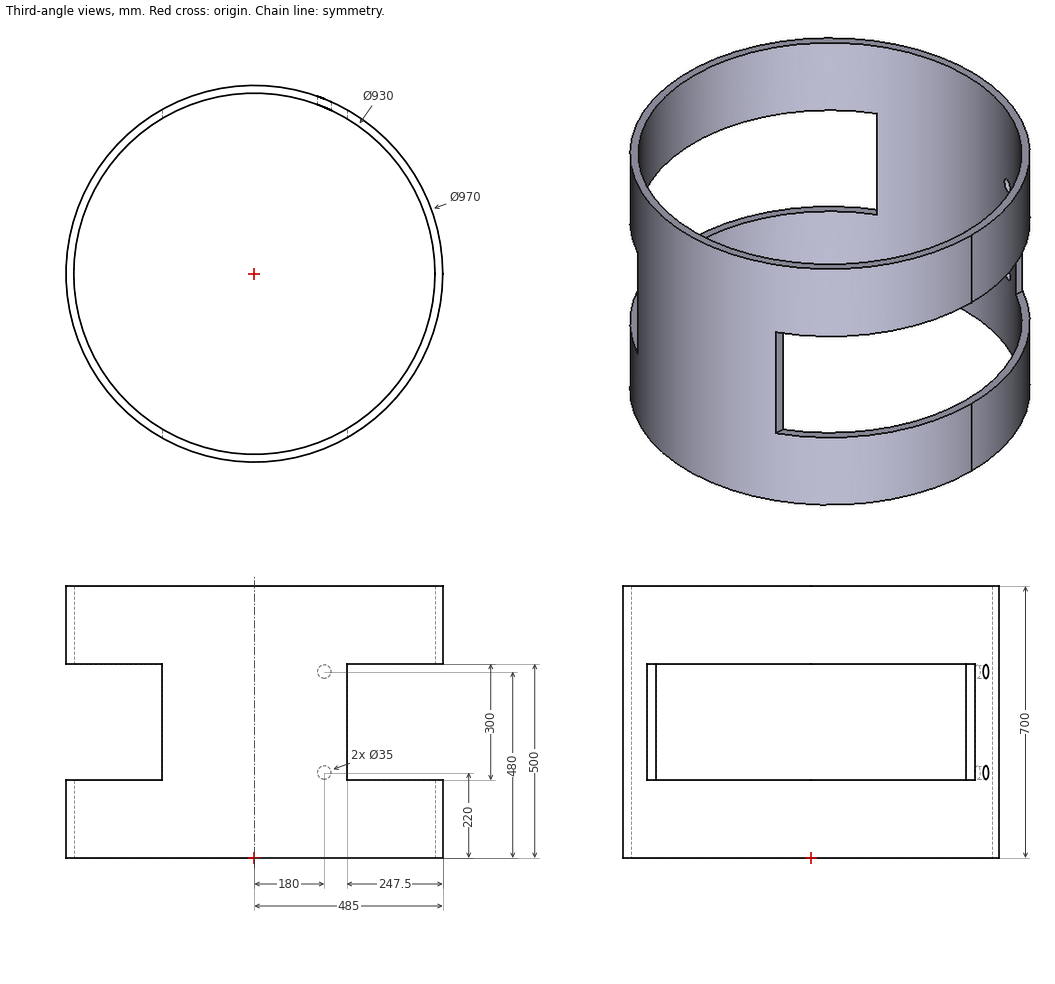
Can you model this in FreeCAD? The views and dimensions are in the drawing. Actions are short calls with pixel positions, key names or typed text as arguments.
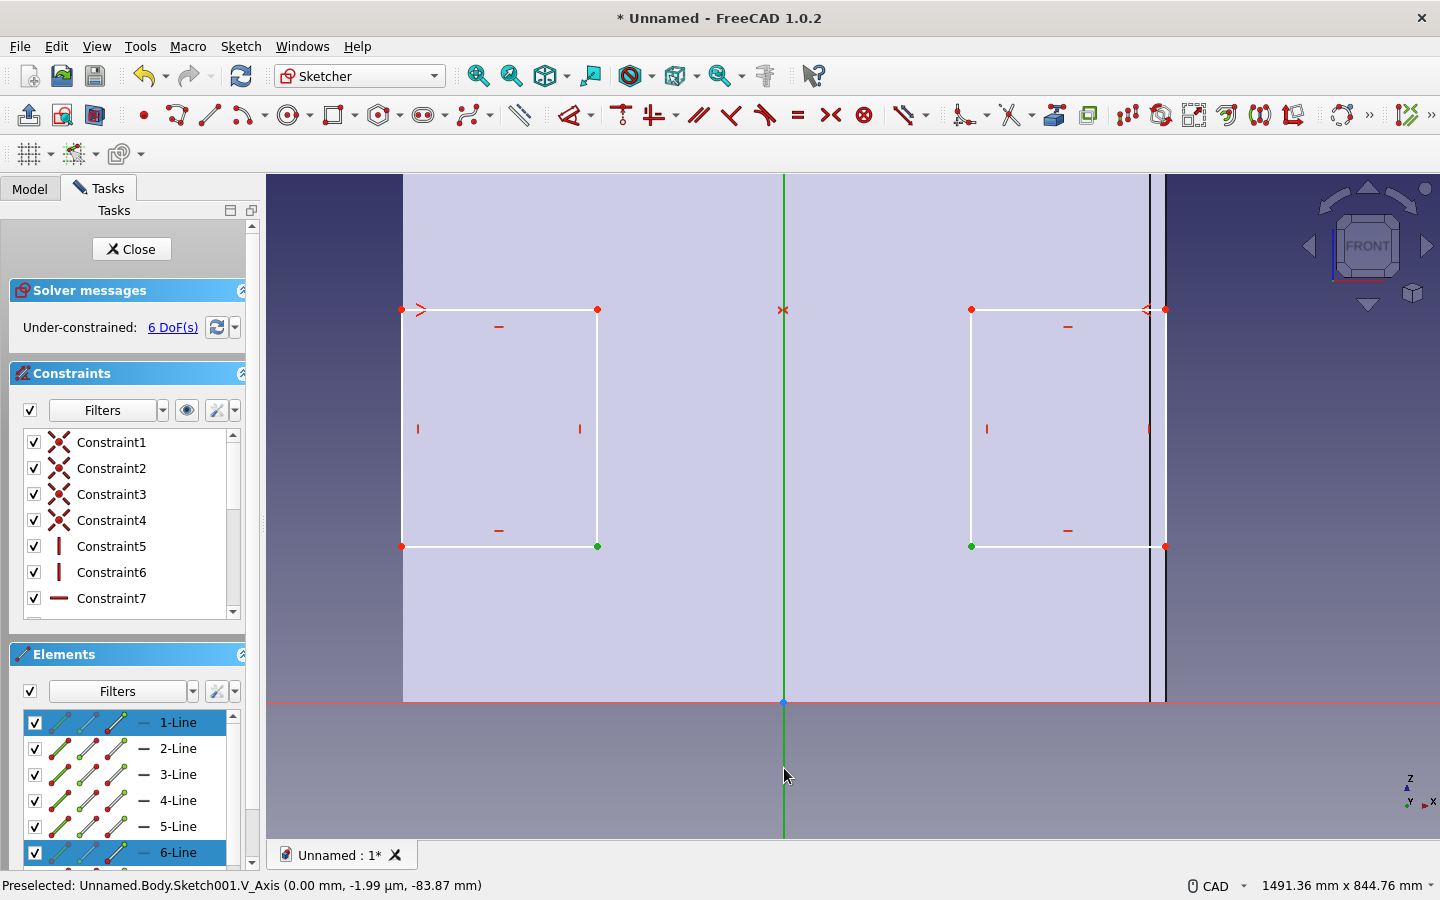
key(s)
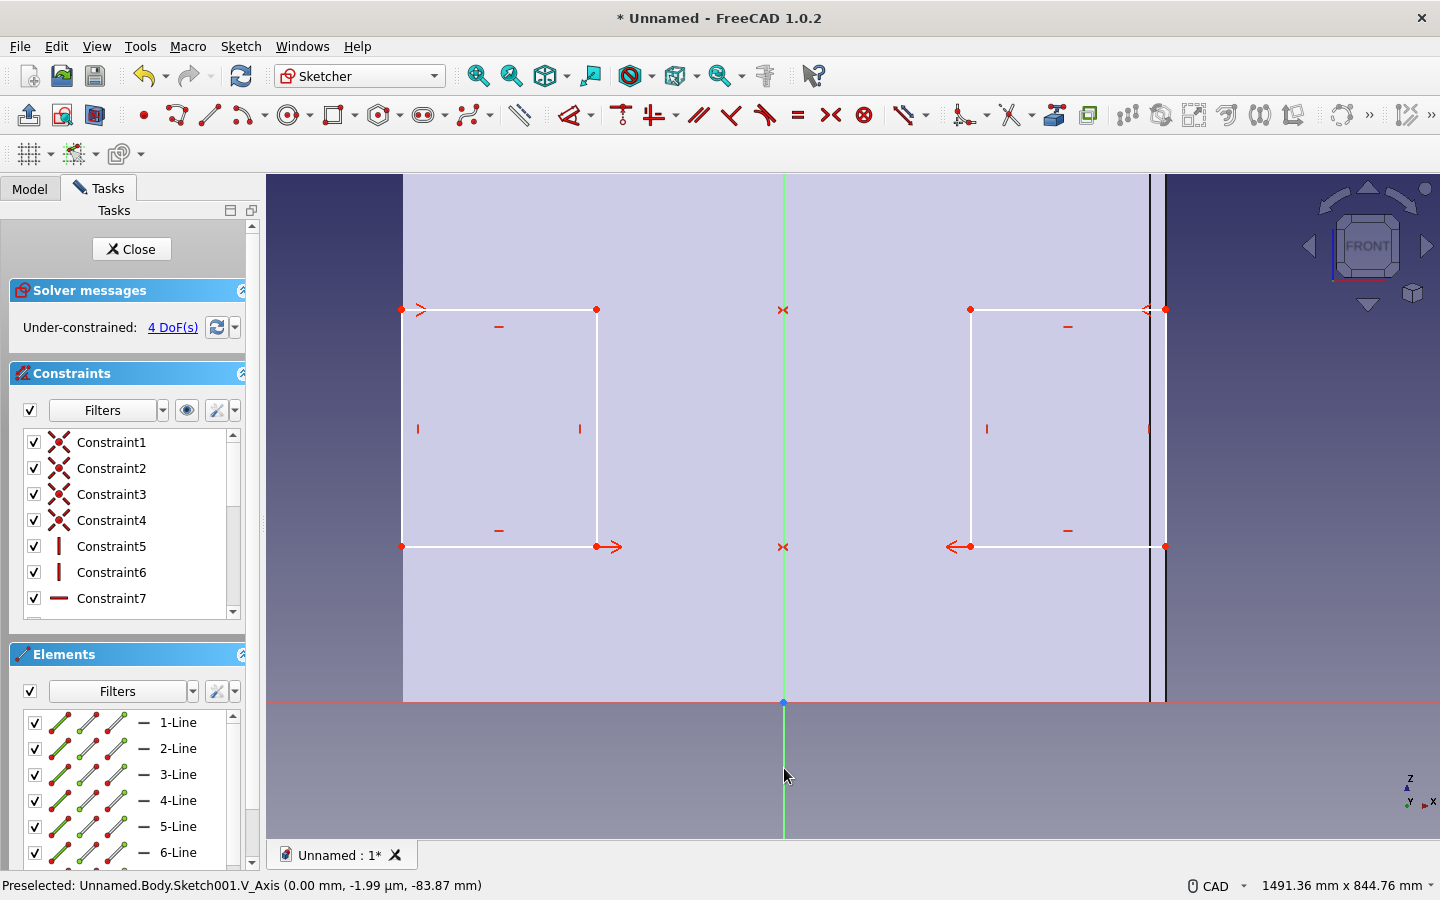
key(d)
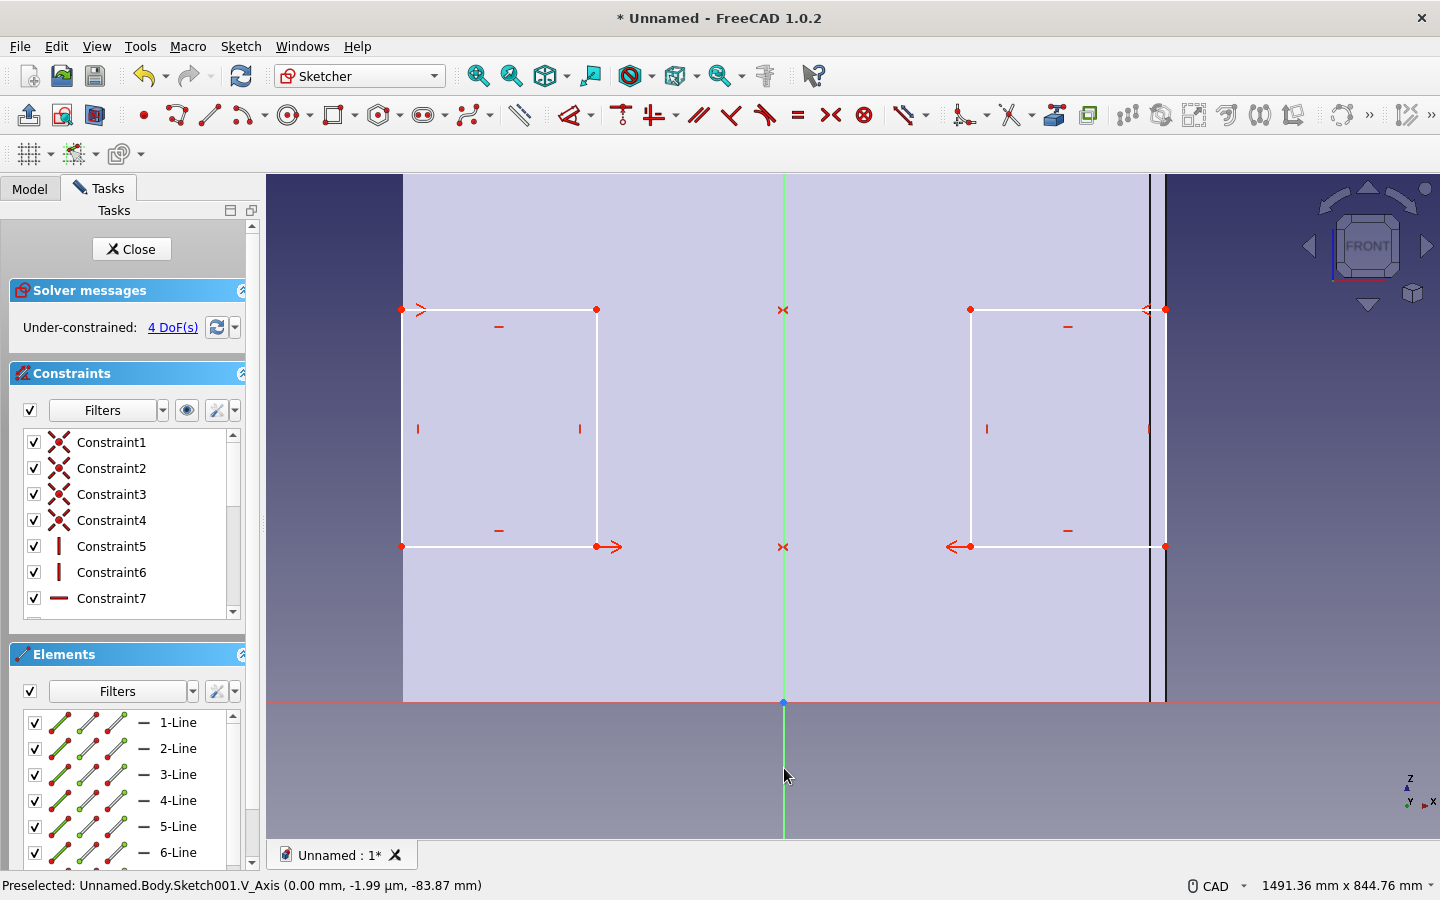
click(971, 381)
click(1005, 429)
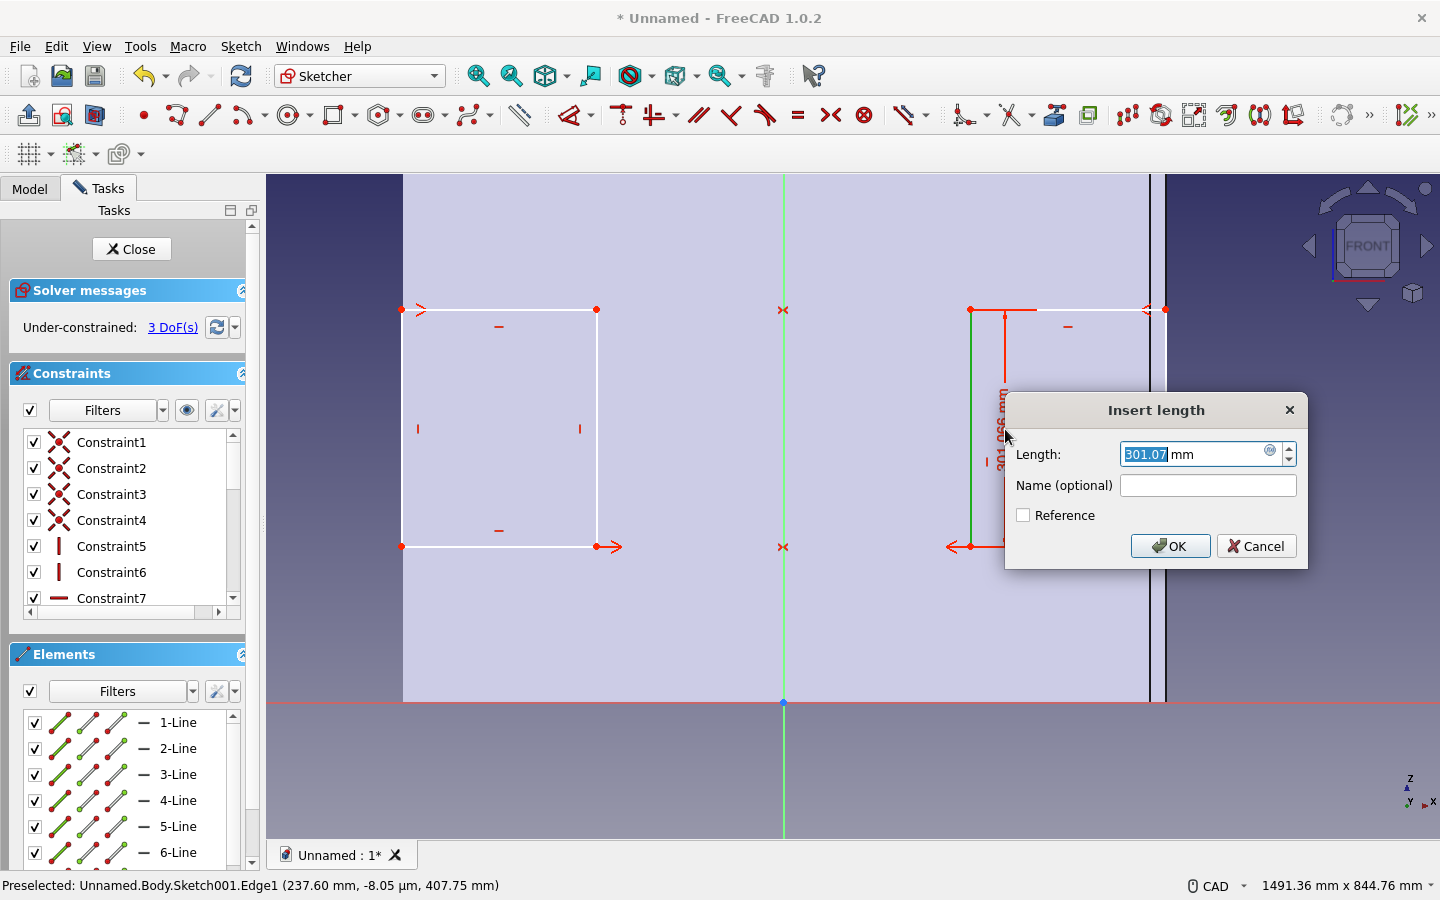
text(300)
key(Return)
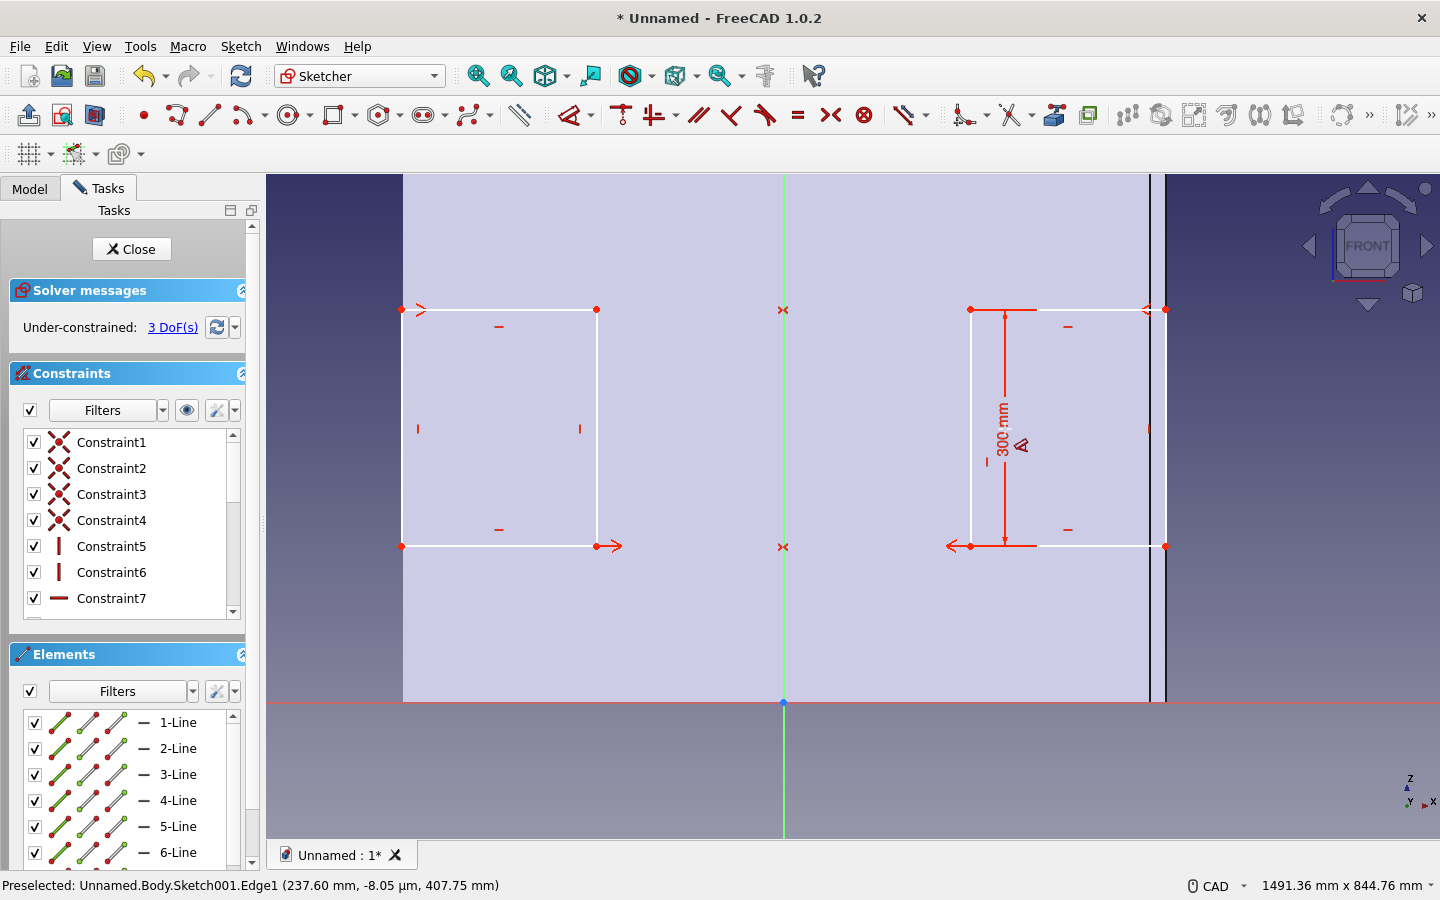
click(971, 310)
click(1005, 506)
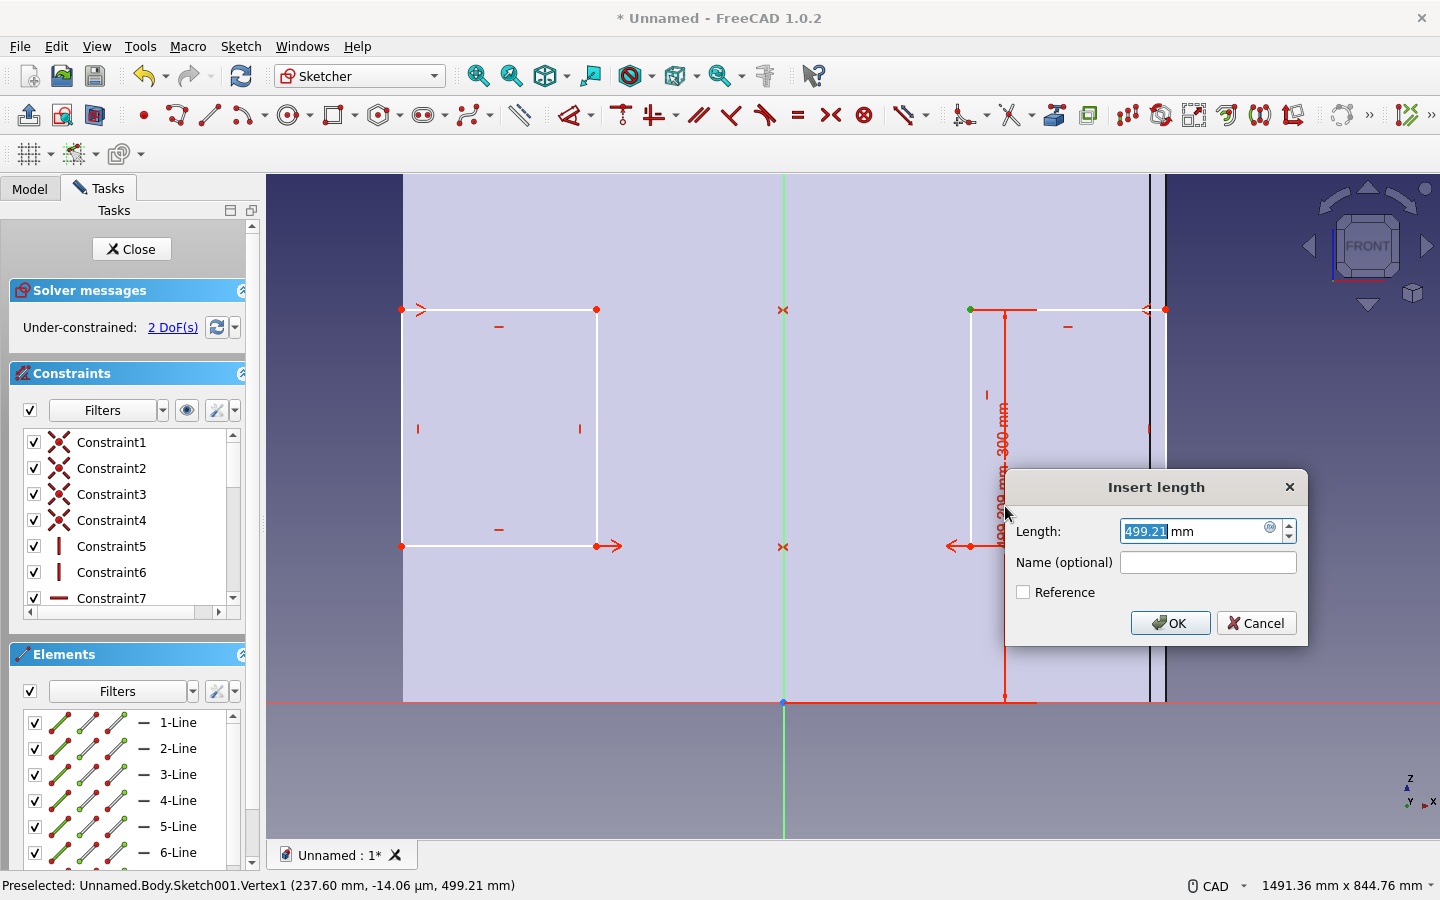
text(500)
key(Return)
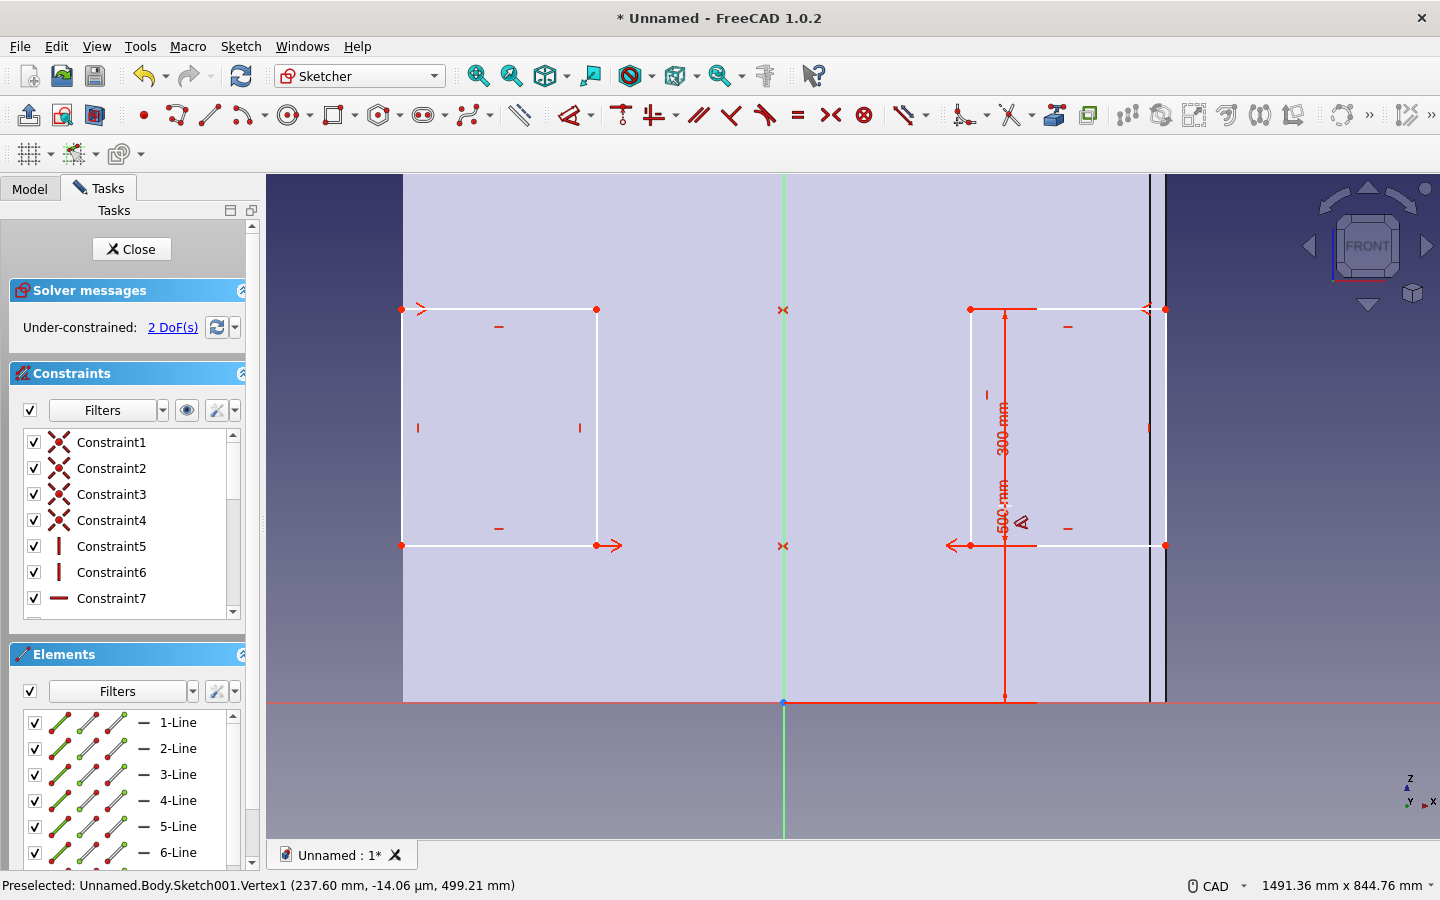
click(1166, 546)
click(975, 737)